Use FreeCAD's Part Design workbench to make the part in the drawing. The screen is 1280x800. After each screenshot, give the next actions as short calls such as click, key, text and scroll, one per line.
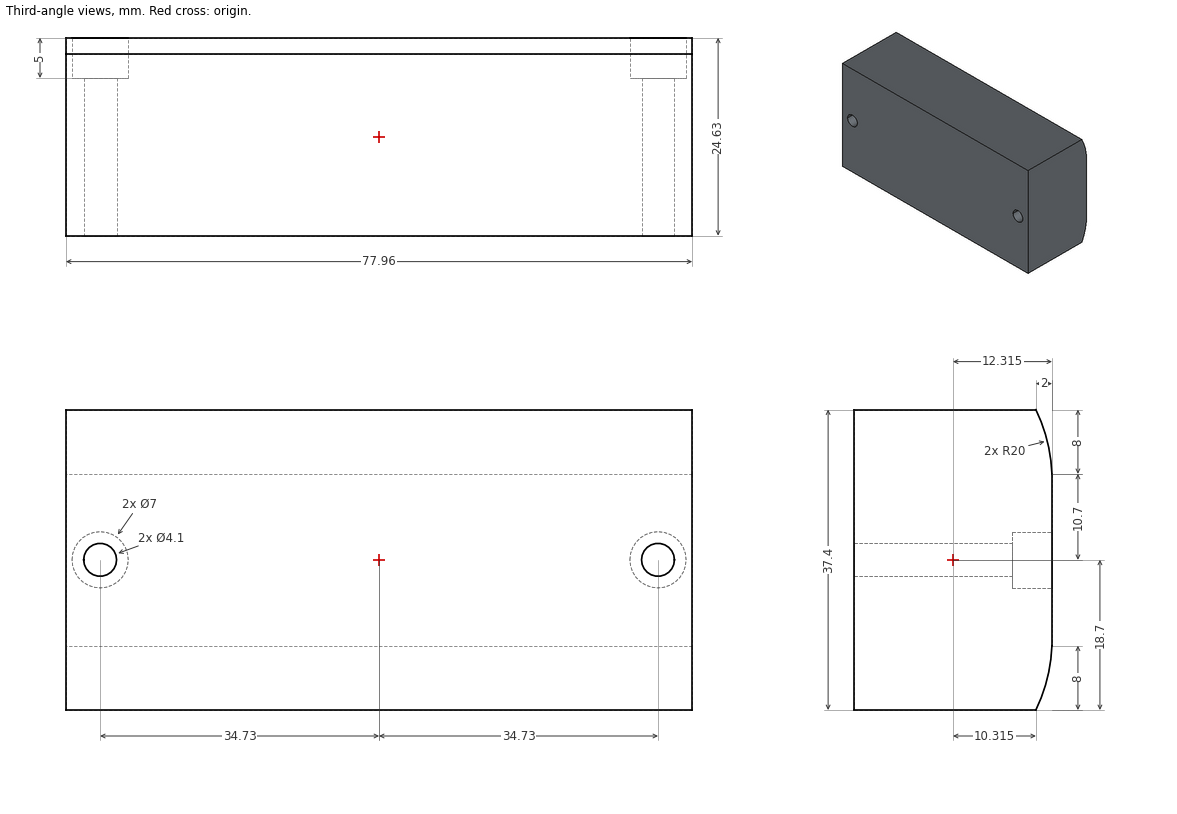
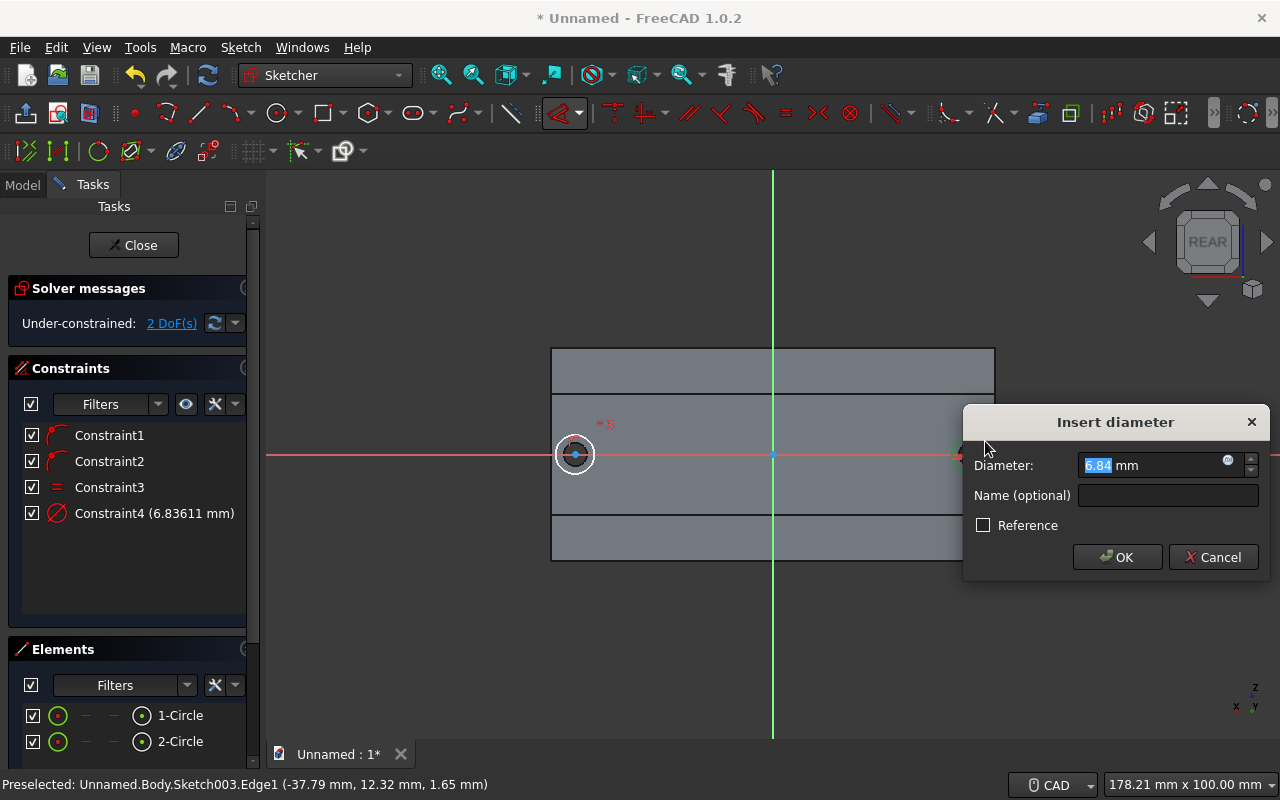
text(7)
key(Return)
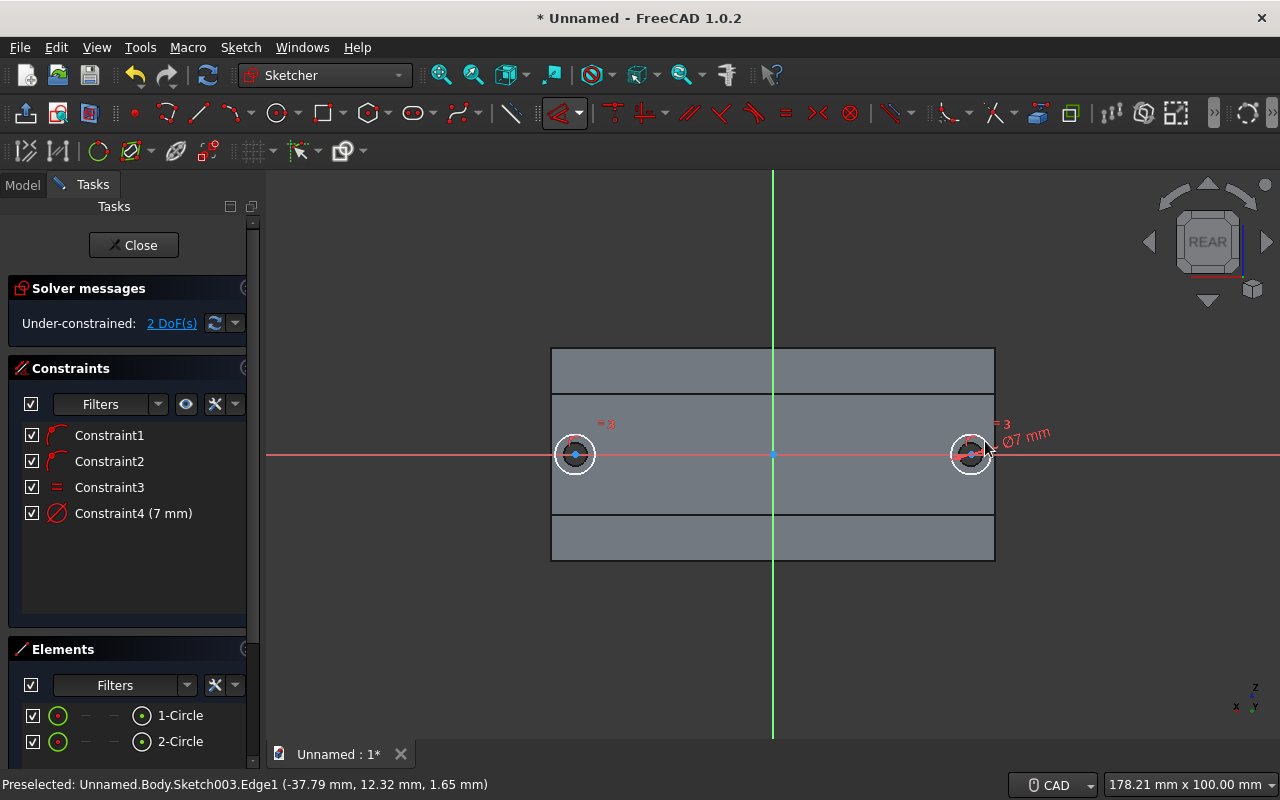
click(971, 455)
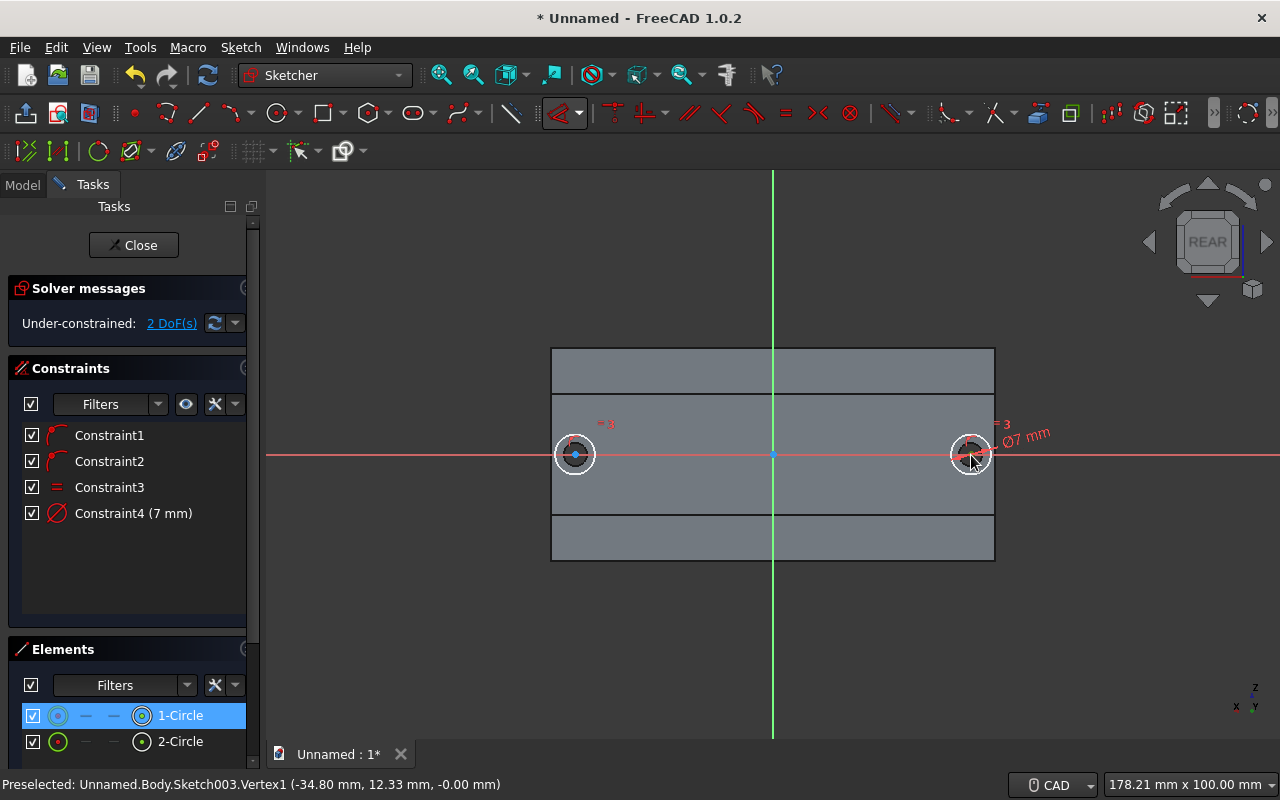
click(582, 114)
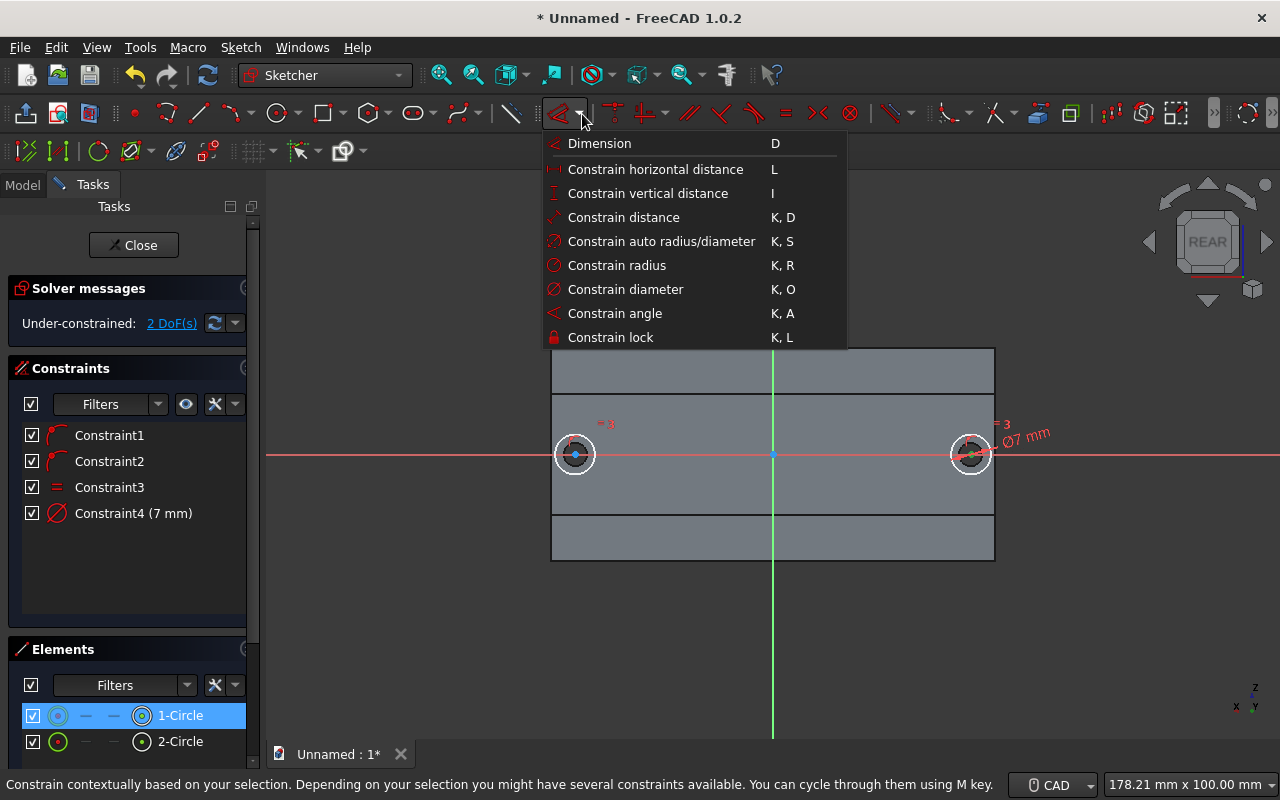
click(695, 169)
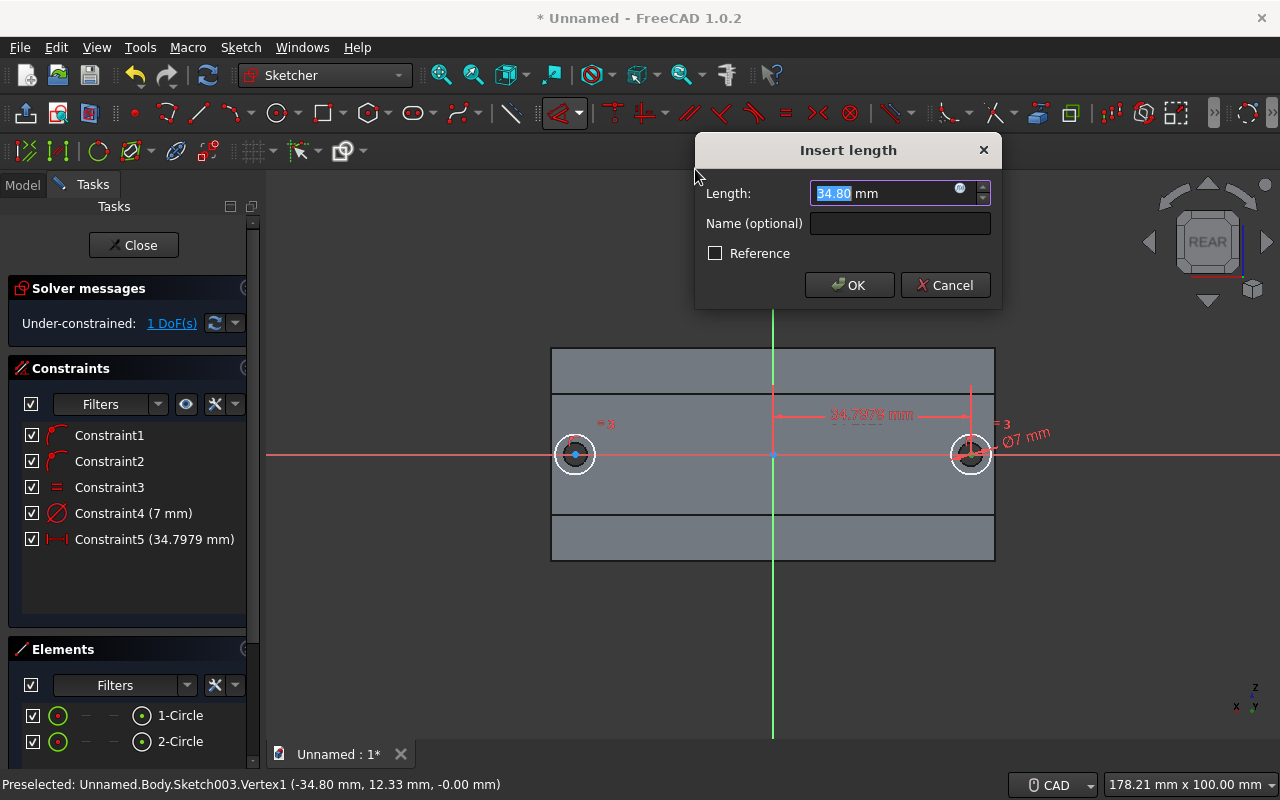
text(34.73)
key(Return)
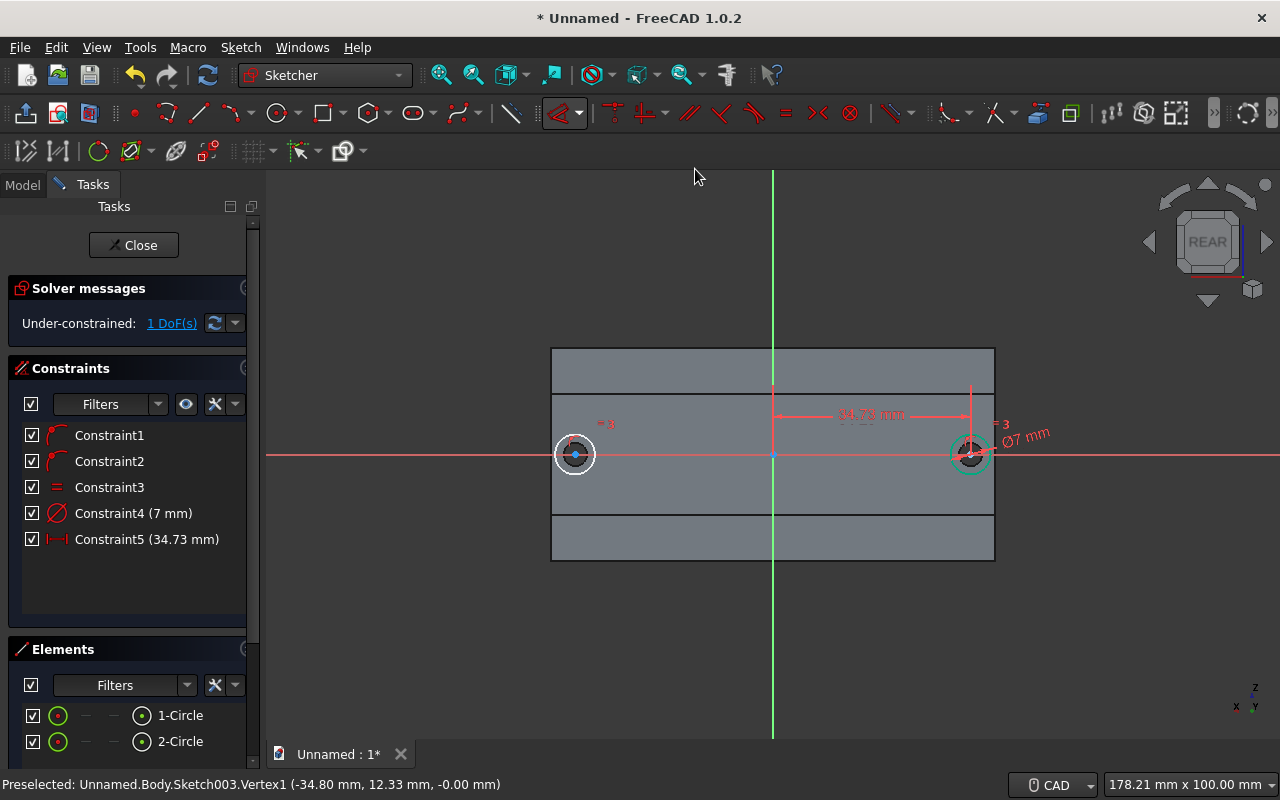
click(575, 455)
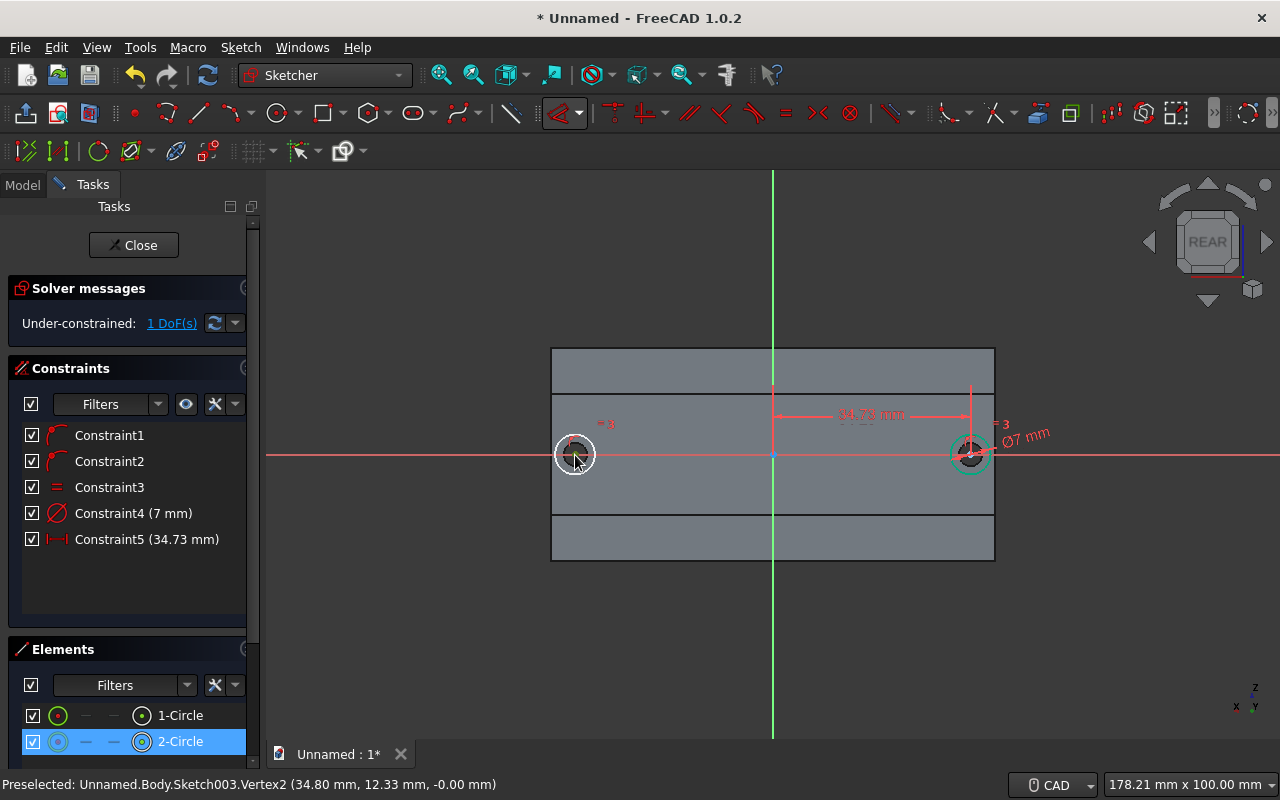
key(l)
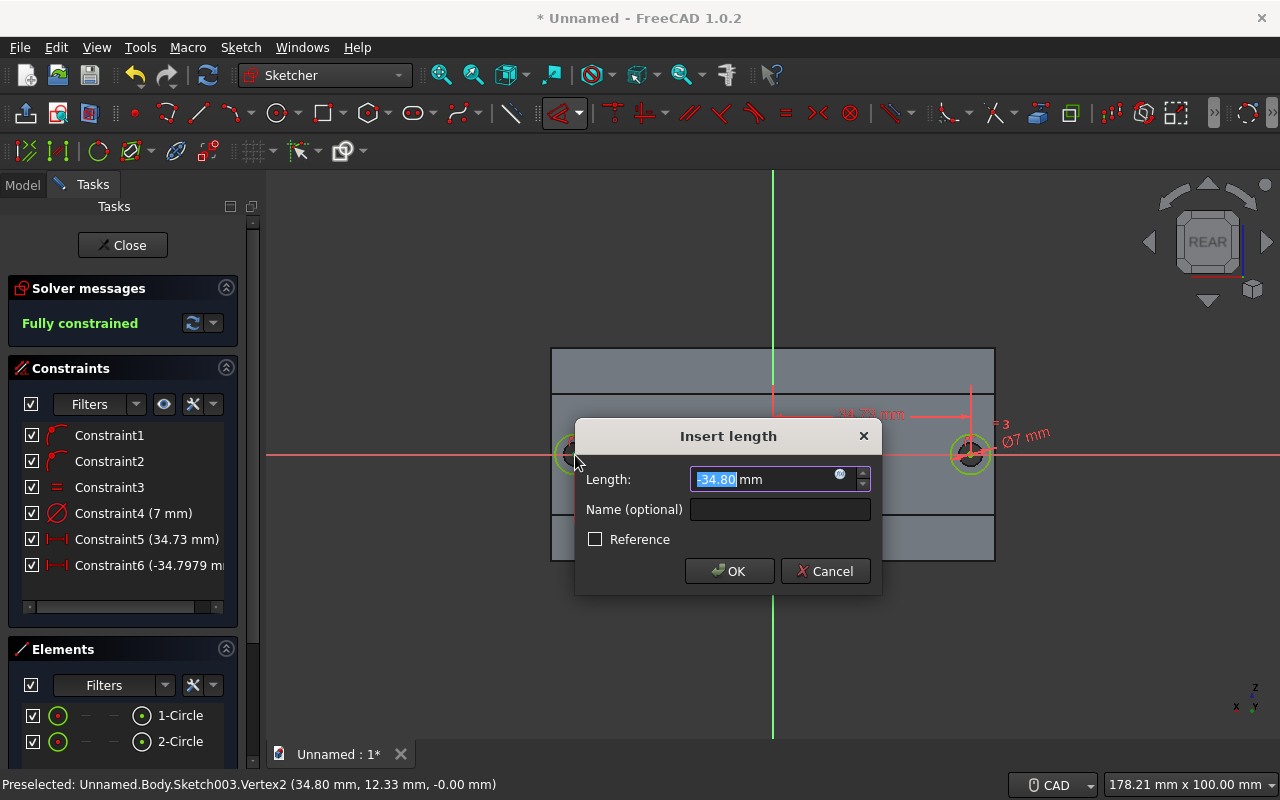
text(-34.73)
key(Return)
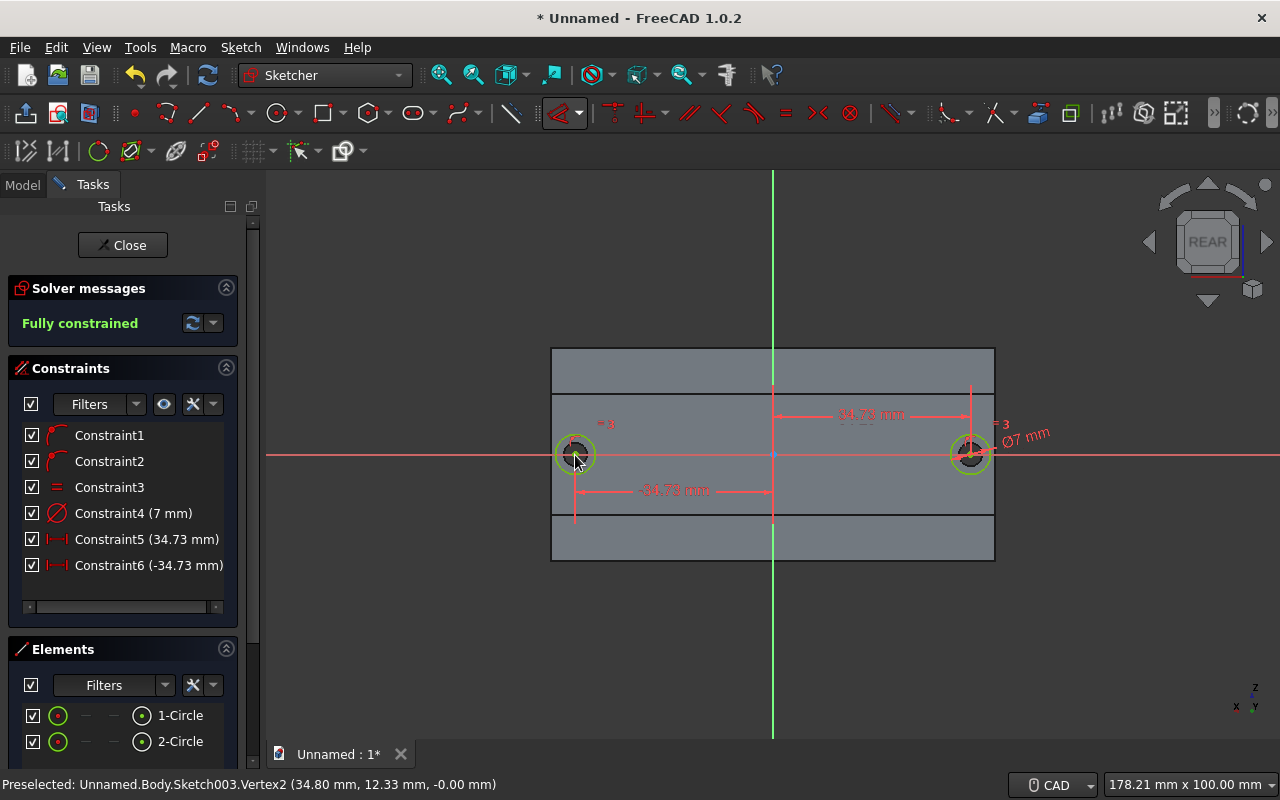
click(123, 245)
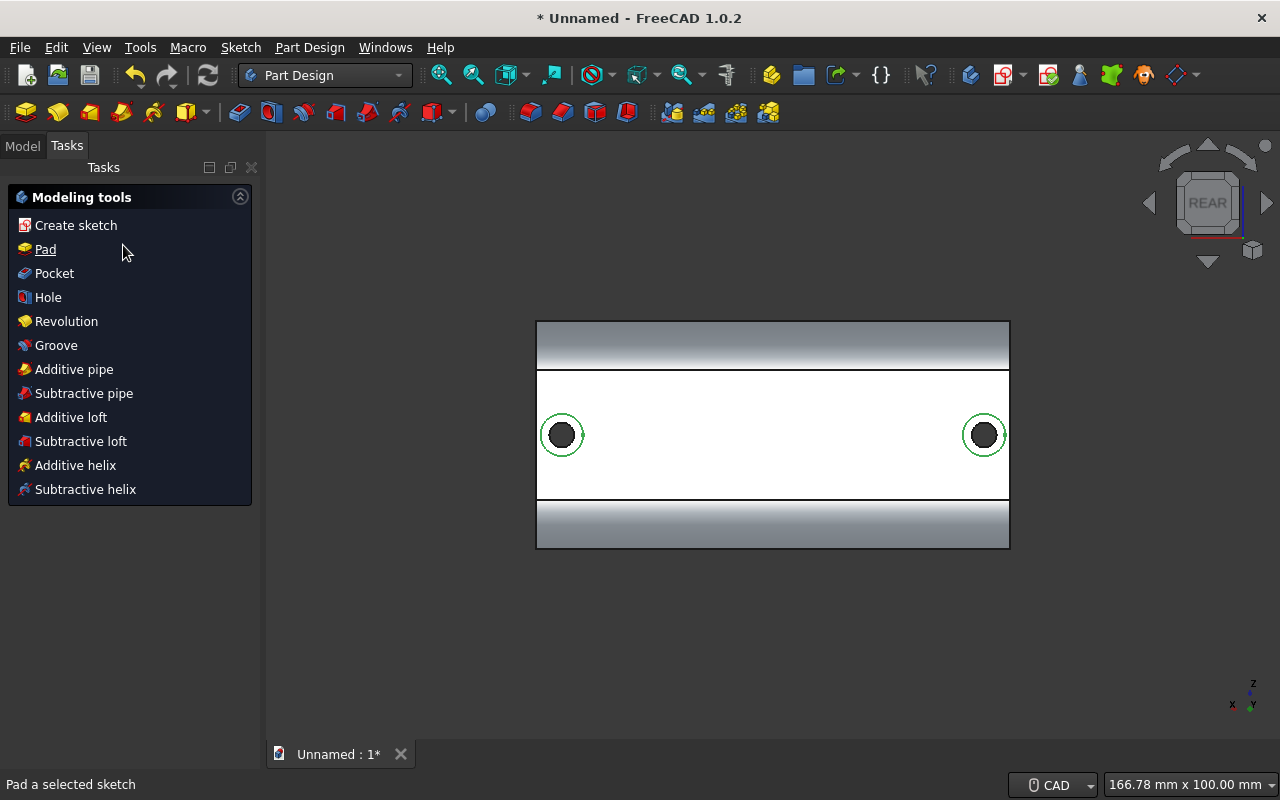
click(240, 112)